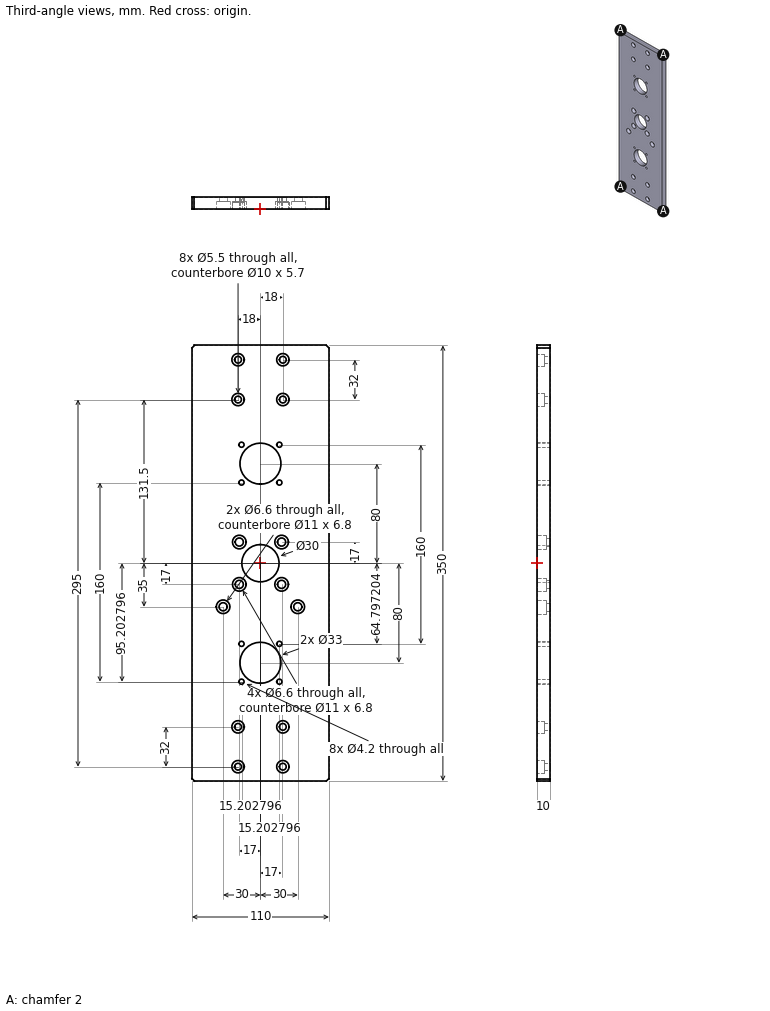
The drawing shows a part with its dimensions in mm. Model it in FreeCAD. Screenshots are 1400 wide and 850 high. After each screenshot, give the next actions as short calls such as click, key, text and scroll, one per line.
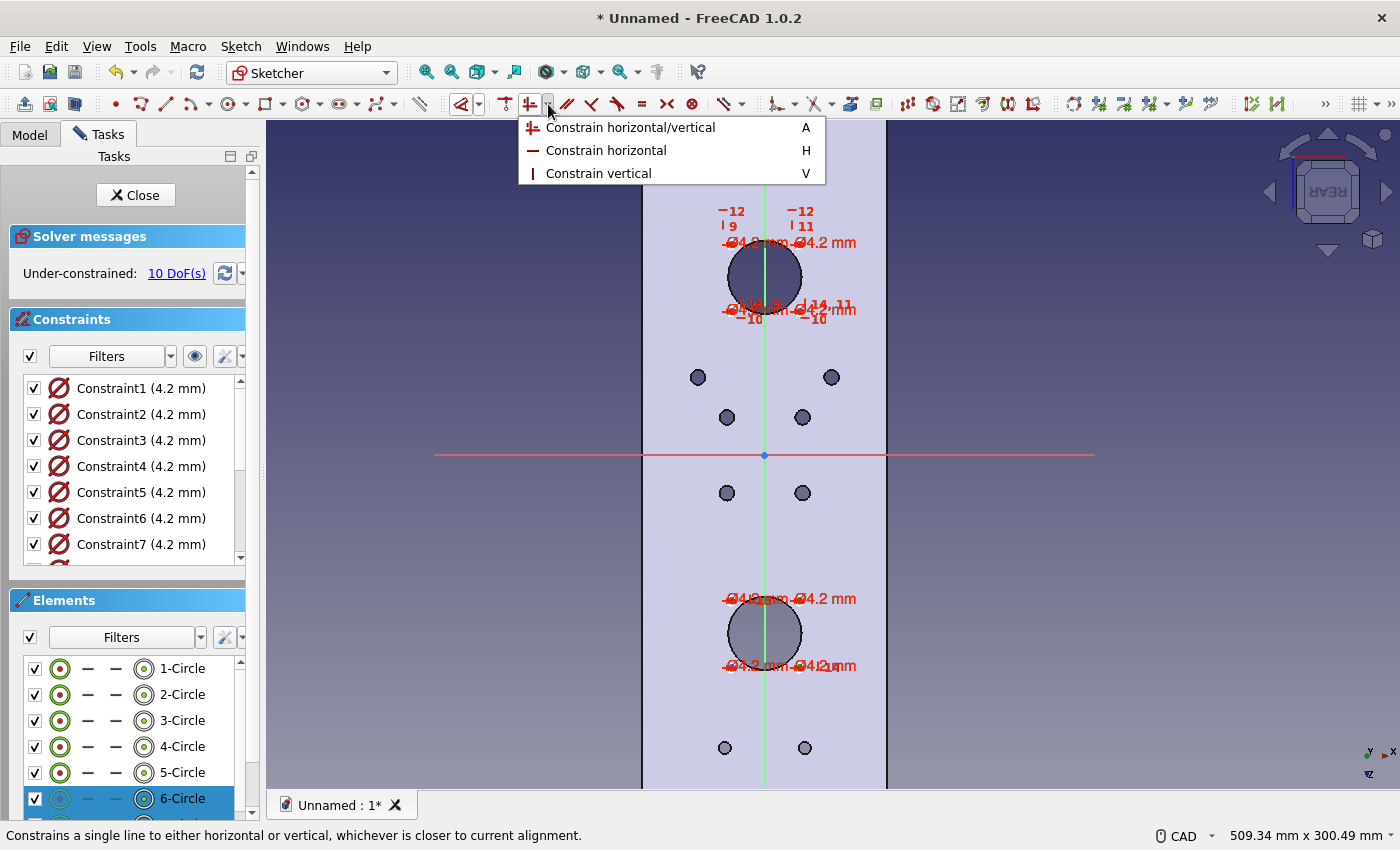
click(672, 174)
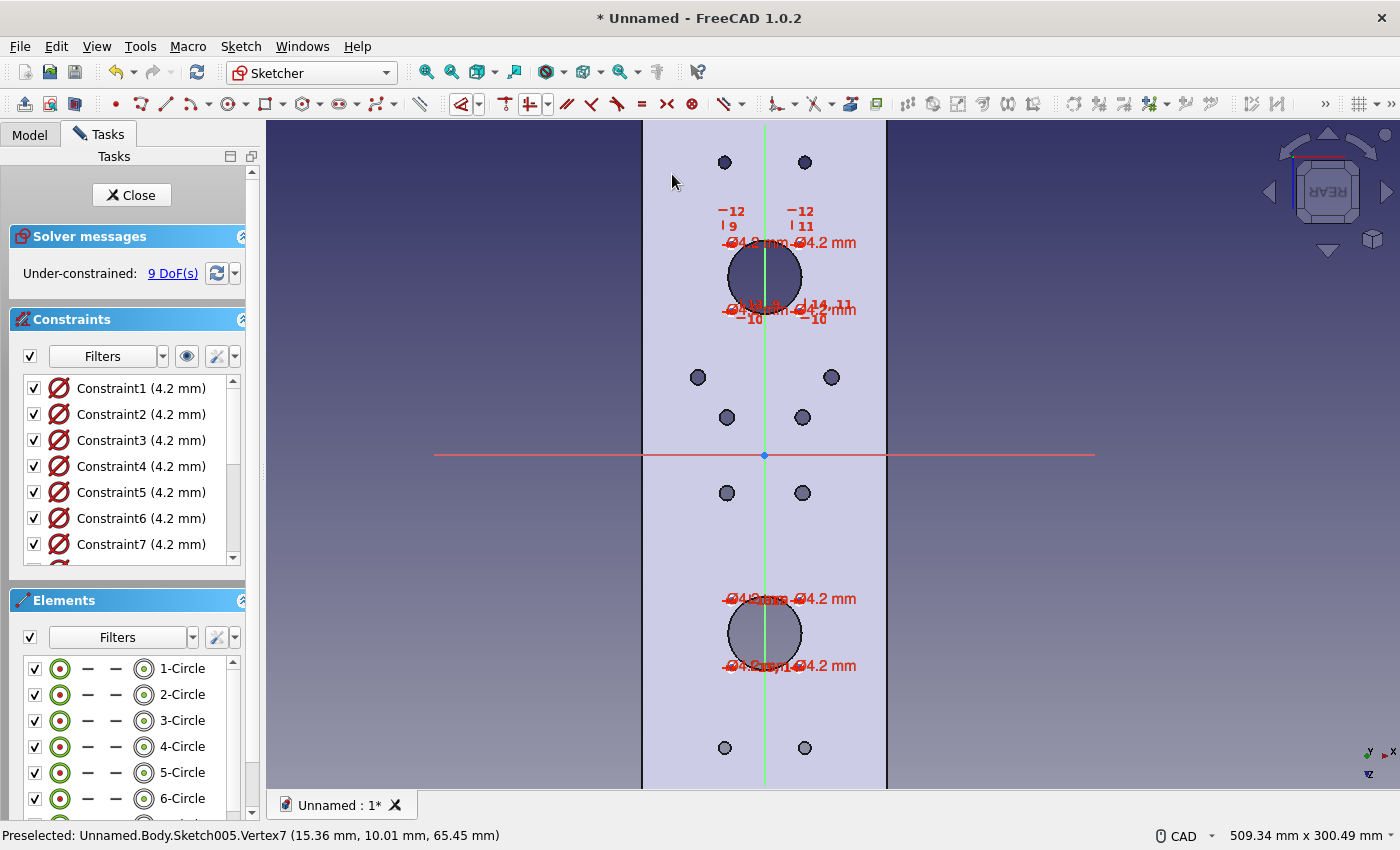
click(731, 601)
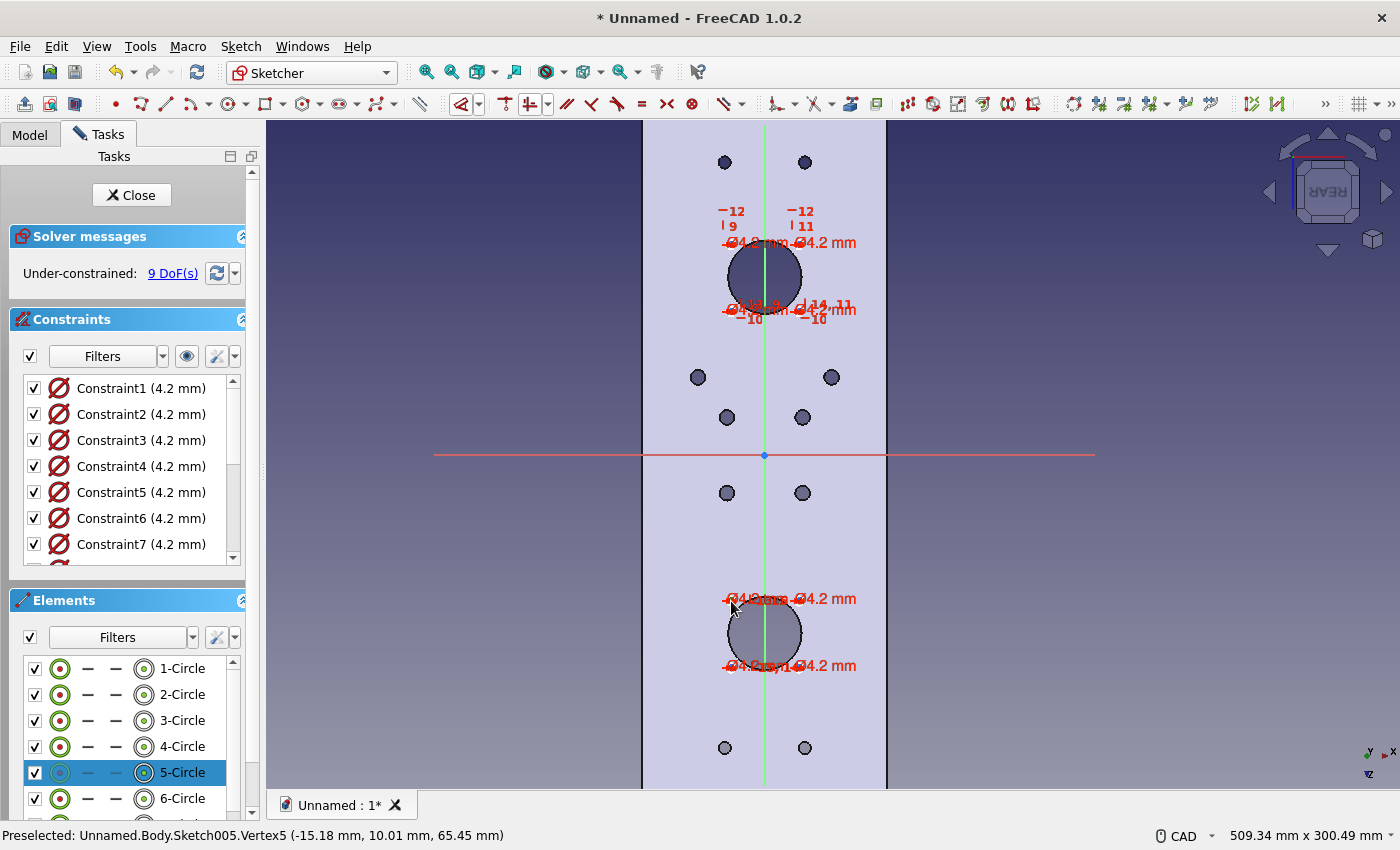
click(799, 601)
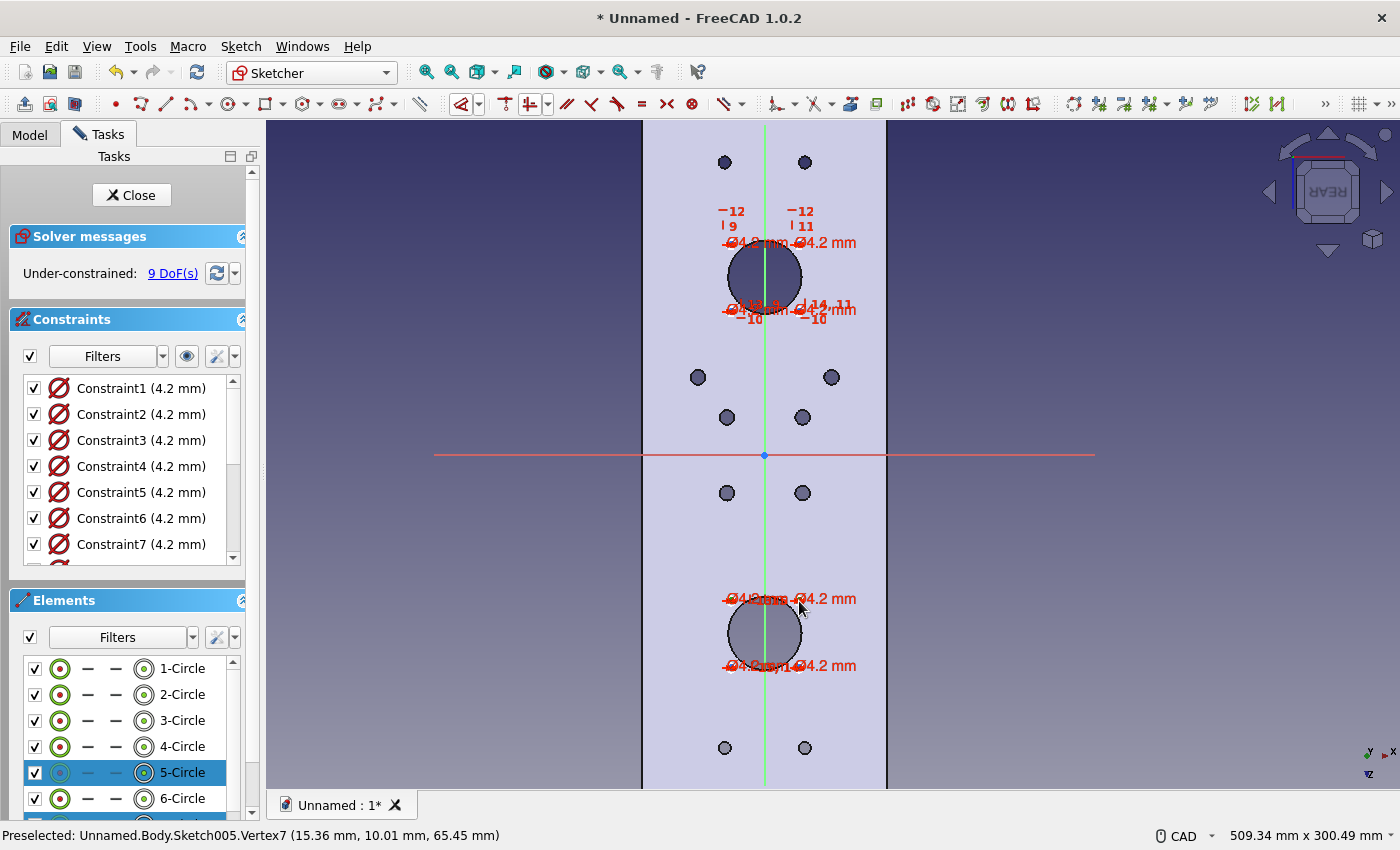
key(h)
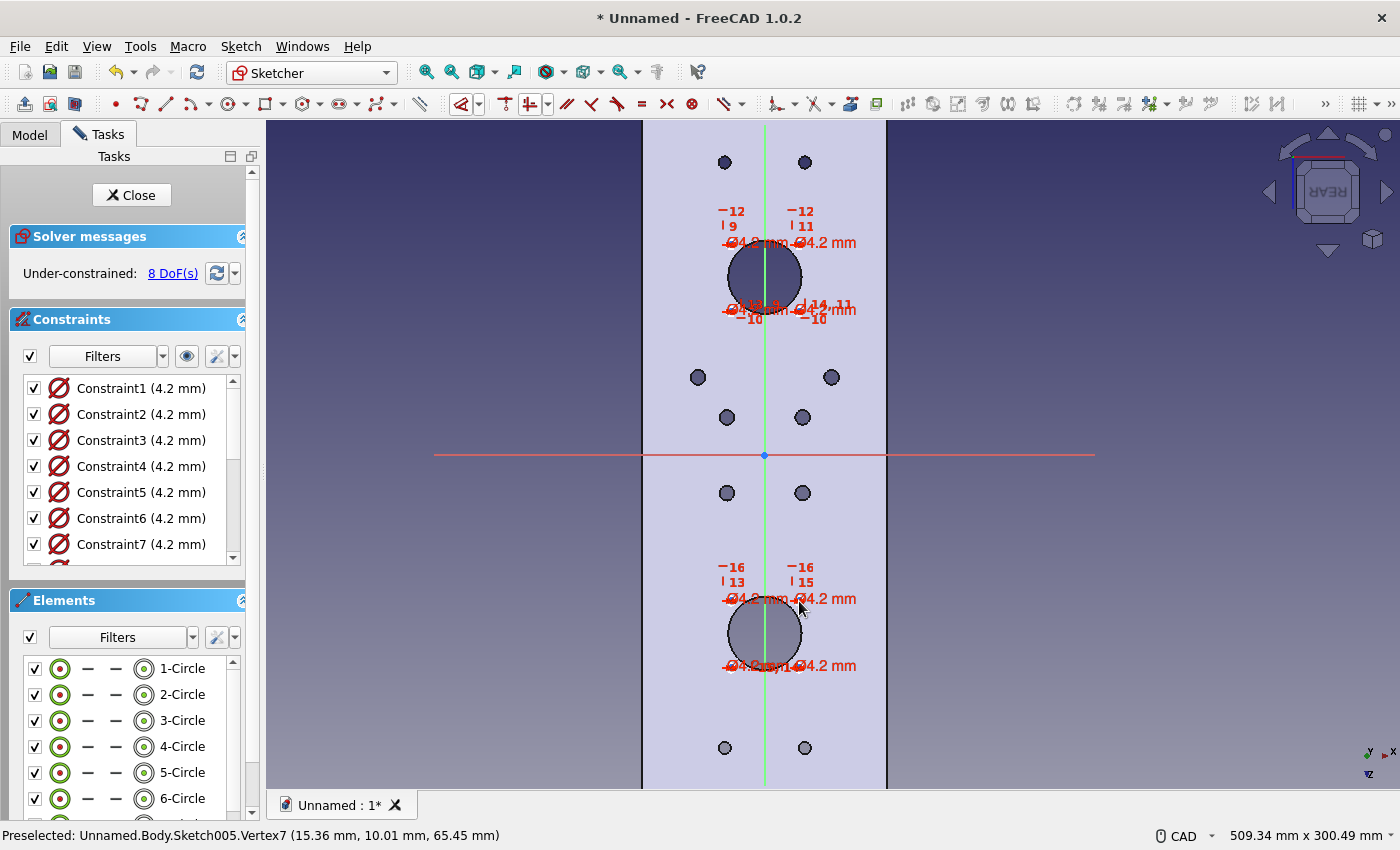
click(731, 601)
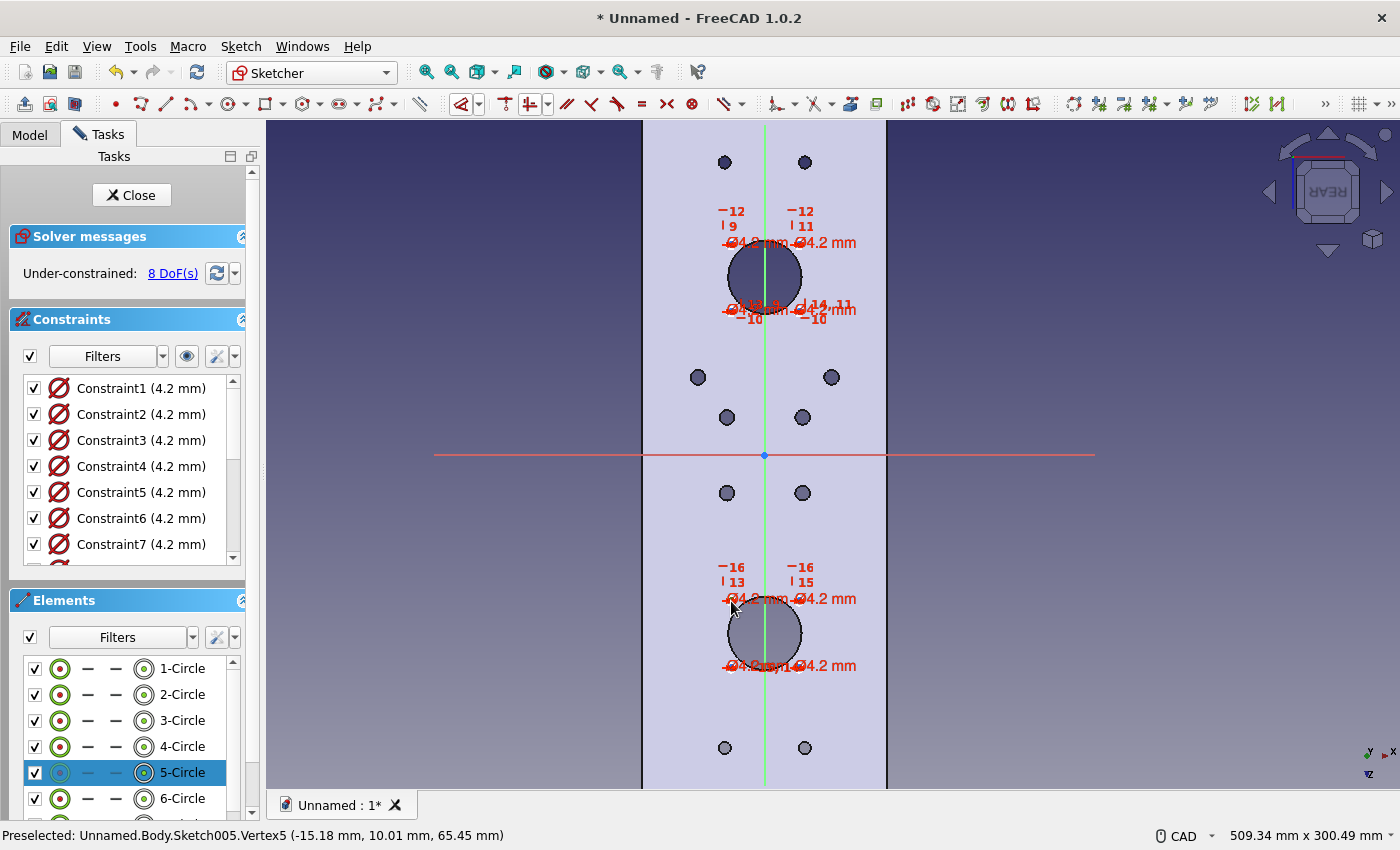
click(731, 668)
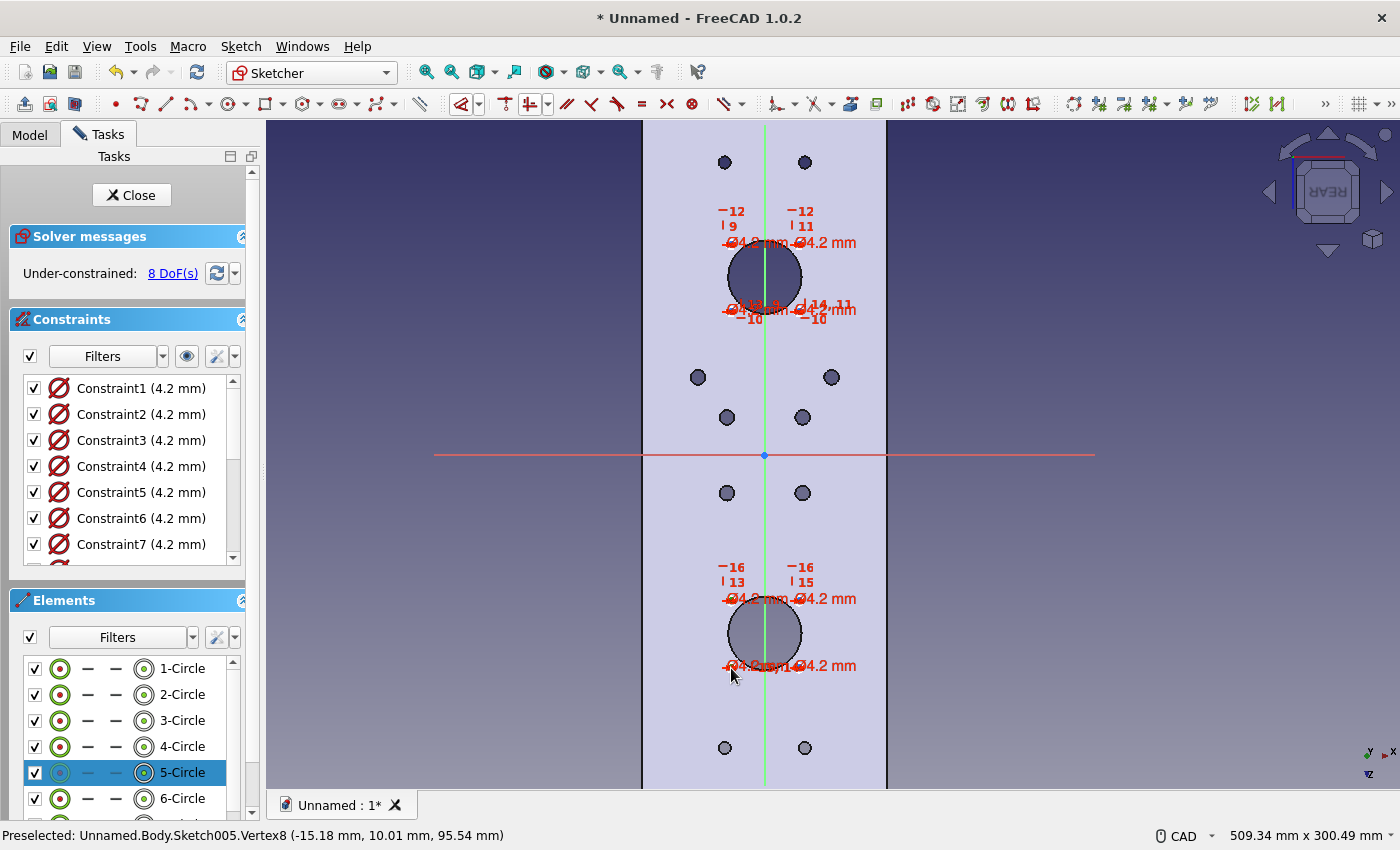
key(v)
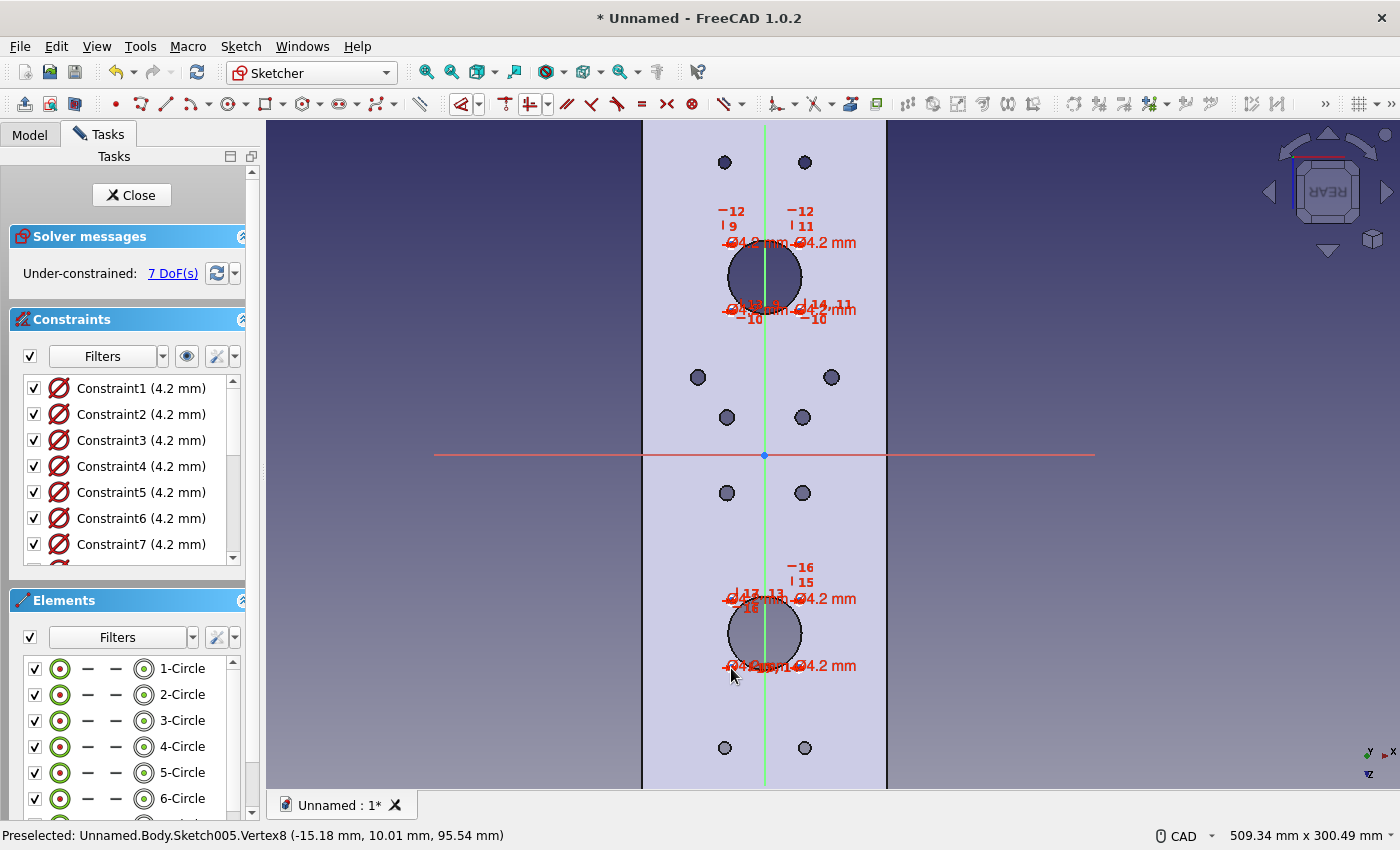
click(799, 668)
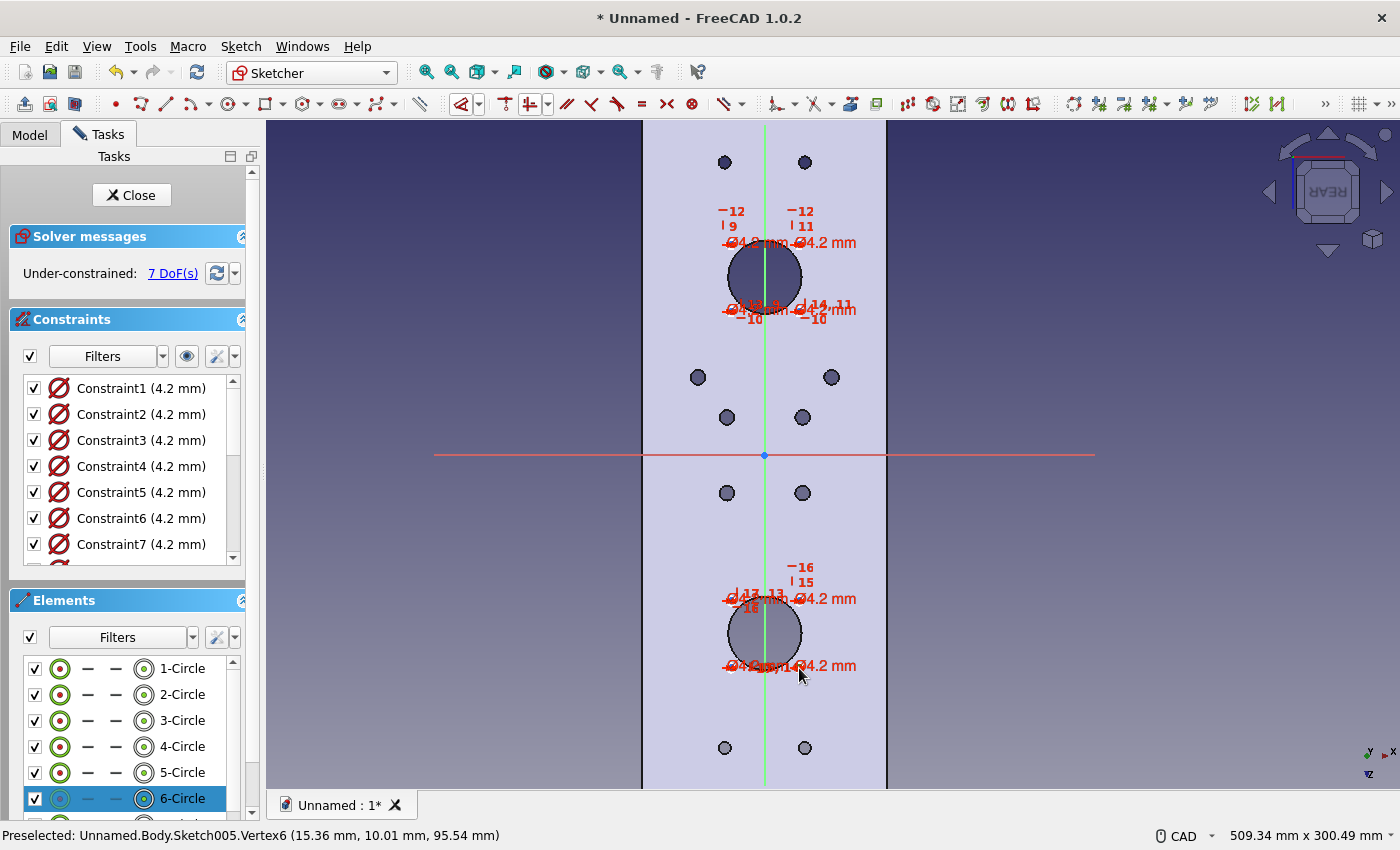
click(731, 668)